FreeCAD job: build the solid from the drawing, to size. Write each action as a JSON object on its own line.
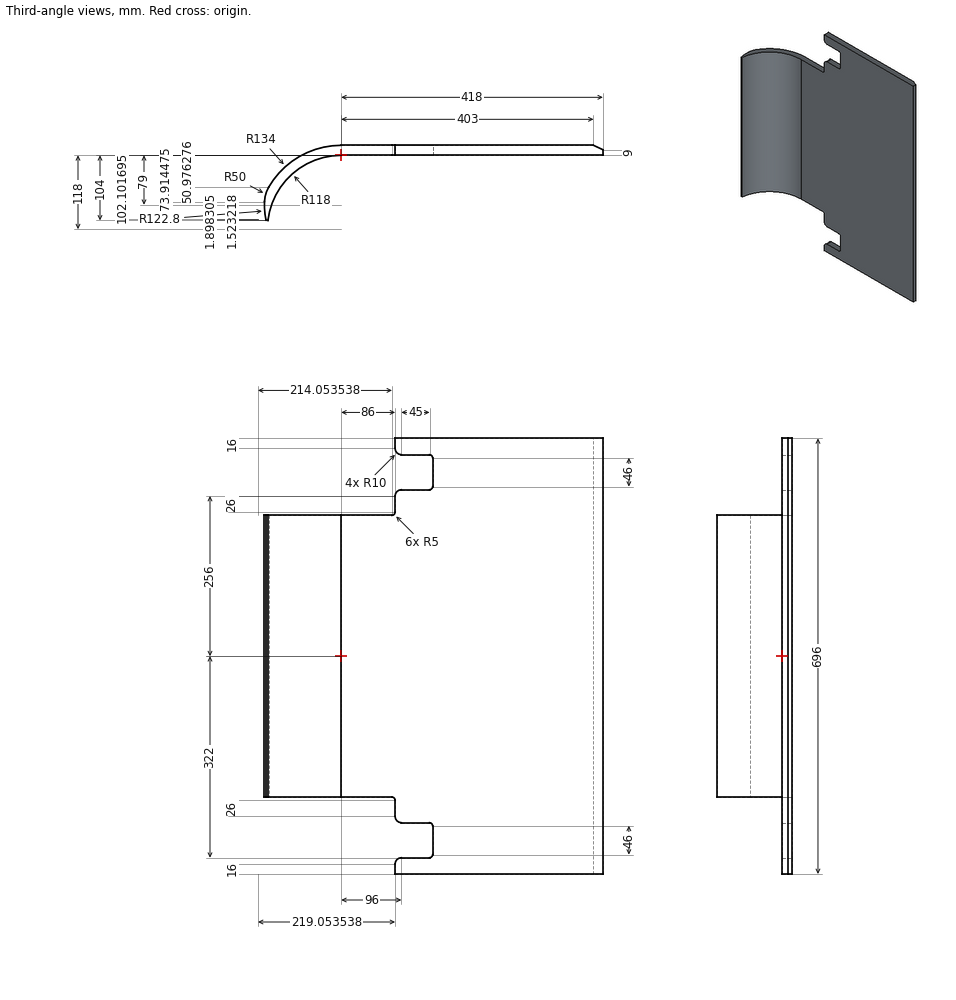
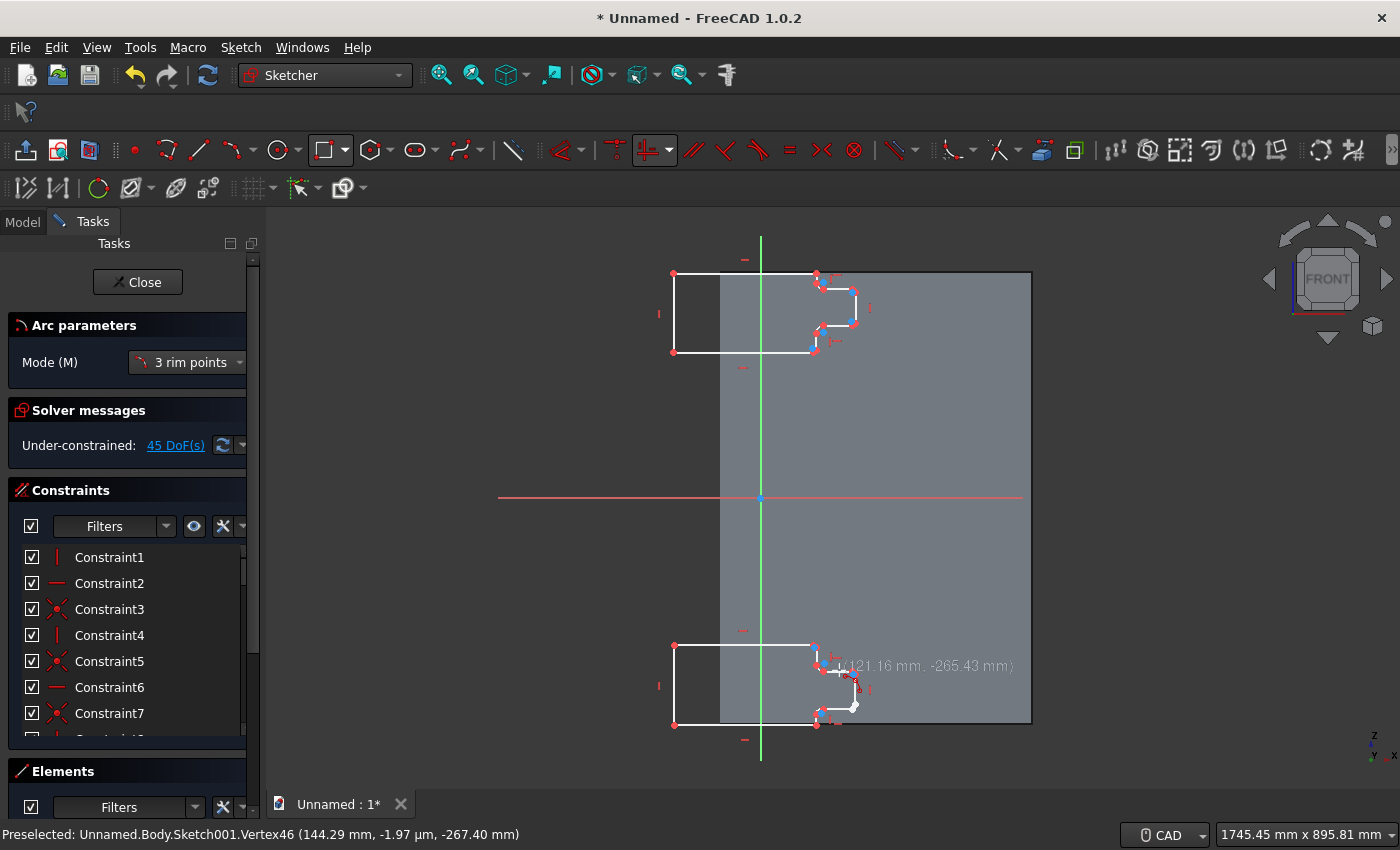
{"action": "scroll", "coordinate": [856, 704], "scroll_direction": "up", "scroll_amount": 7}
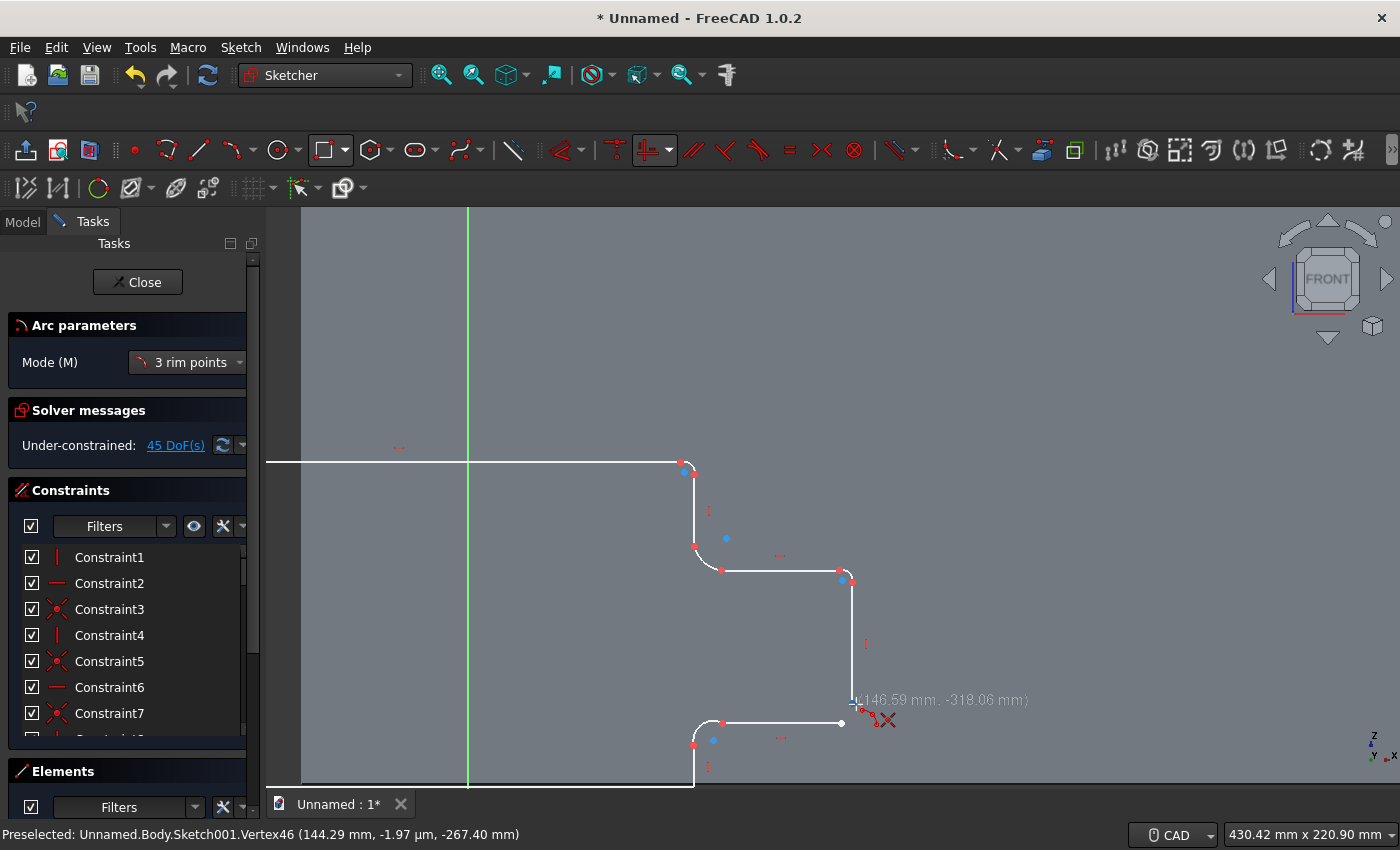
{"action": "left_click", "coordinate": [852, 704]}
{"action": "left_click", "coordinate": [841, 723]}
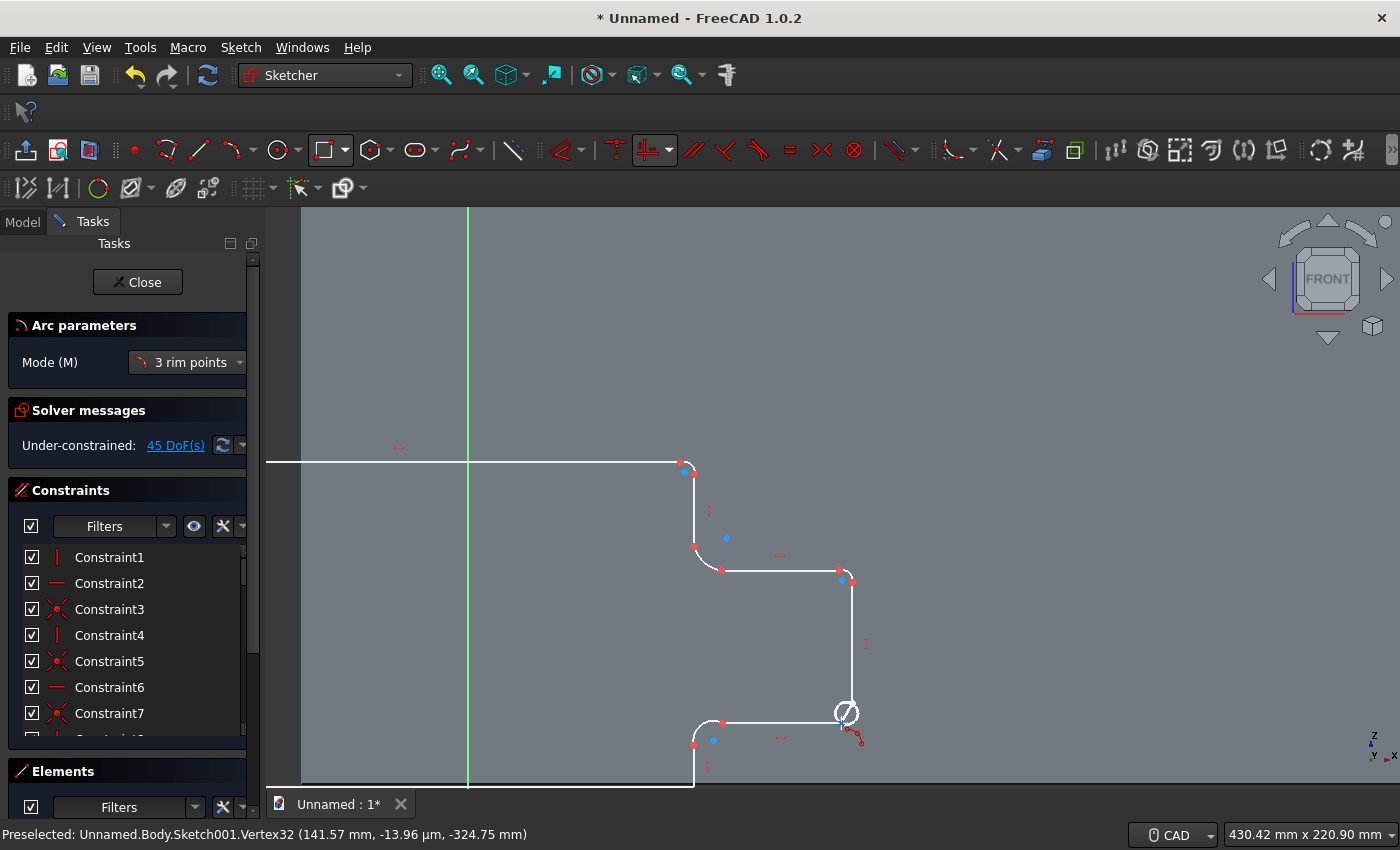
{"action": "scroll", "coordinate": [849, 712], "scroll_direction": "up", "scroll_amount": 8}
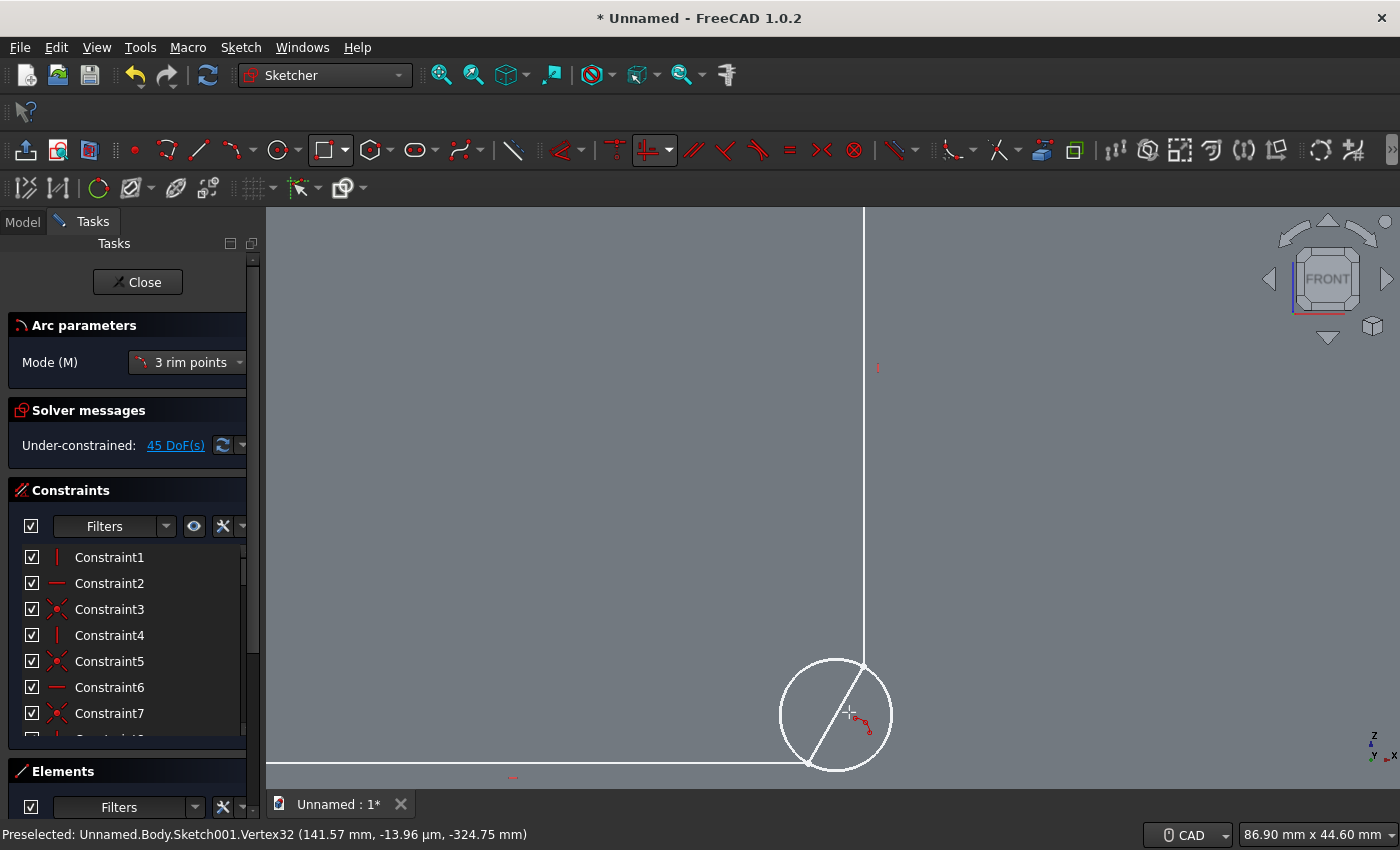
{"action": "left_click", "coordinate": [847, 708]}
{"action": "key", "text": "Escape"}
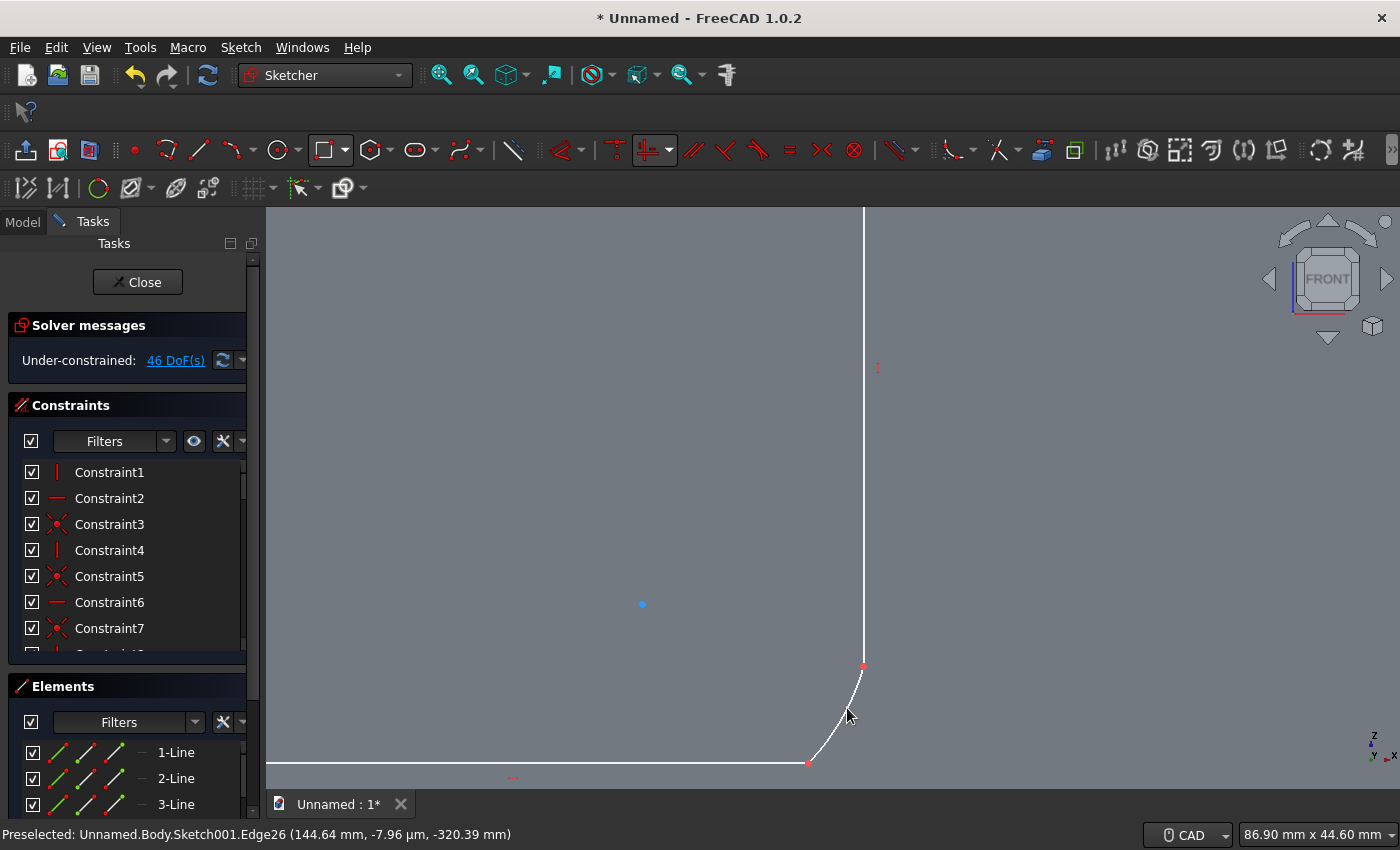
{"action": "scroll", "coordinate": [855, 706], "scroll_direction": "down", "scroll_amount": 15}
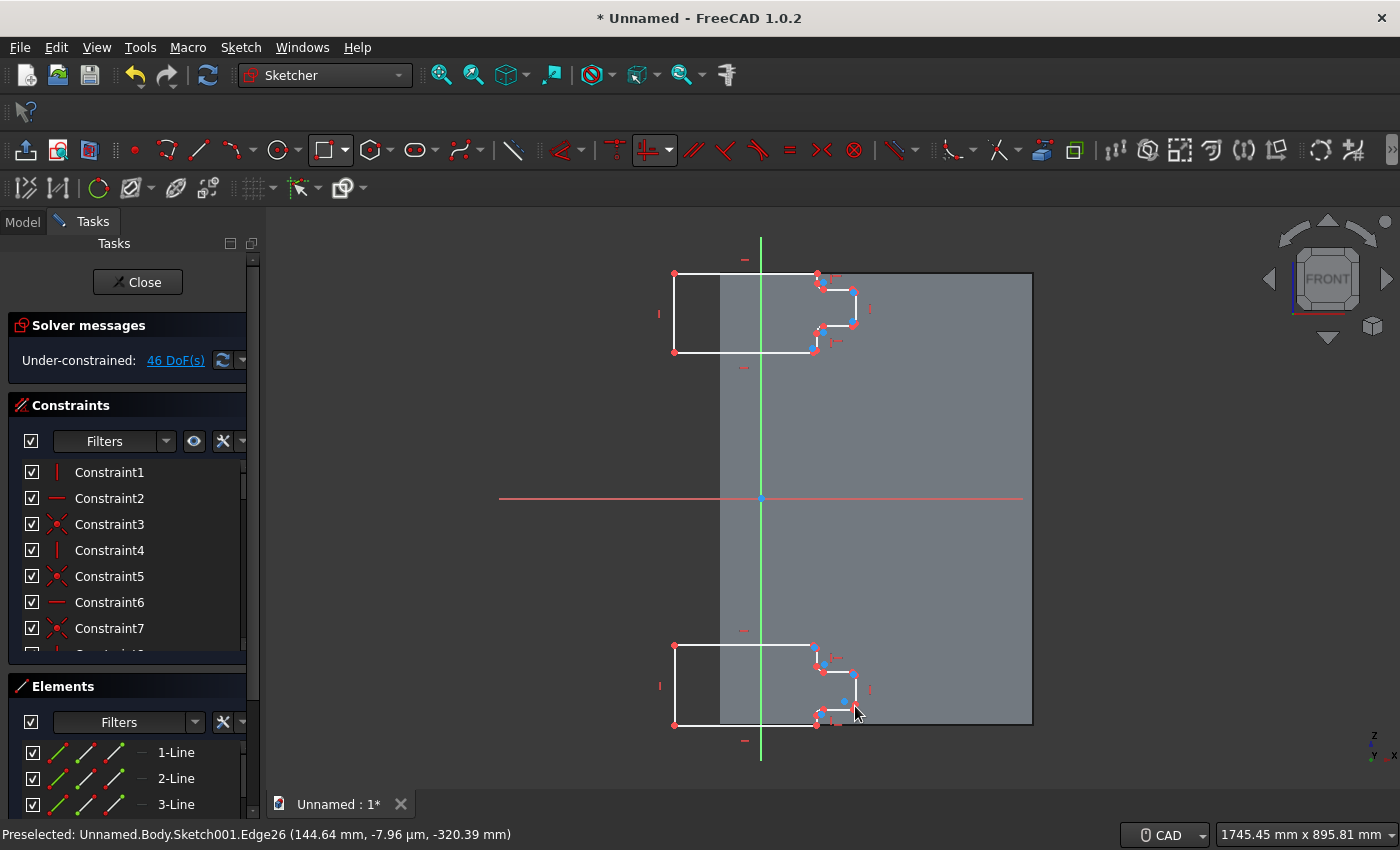
{"action": "scroll", "coordinate": [817, 339], "scroll_direction": "up", "scroll_amount": 5}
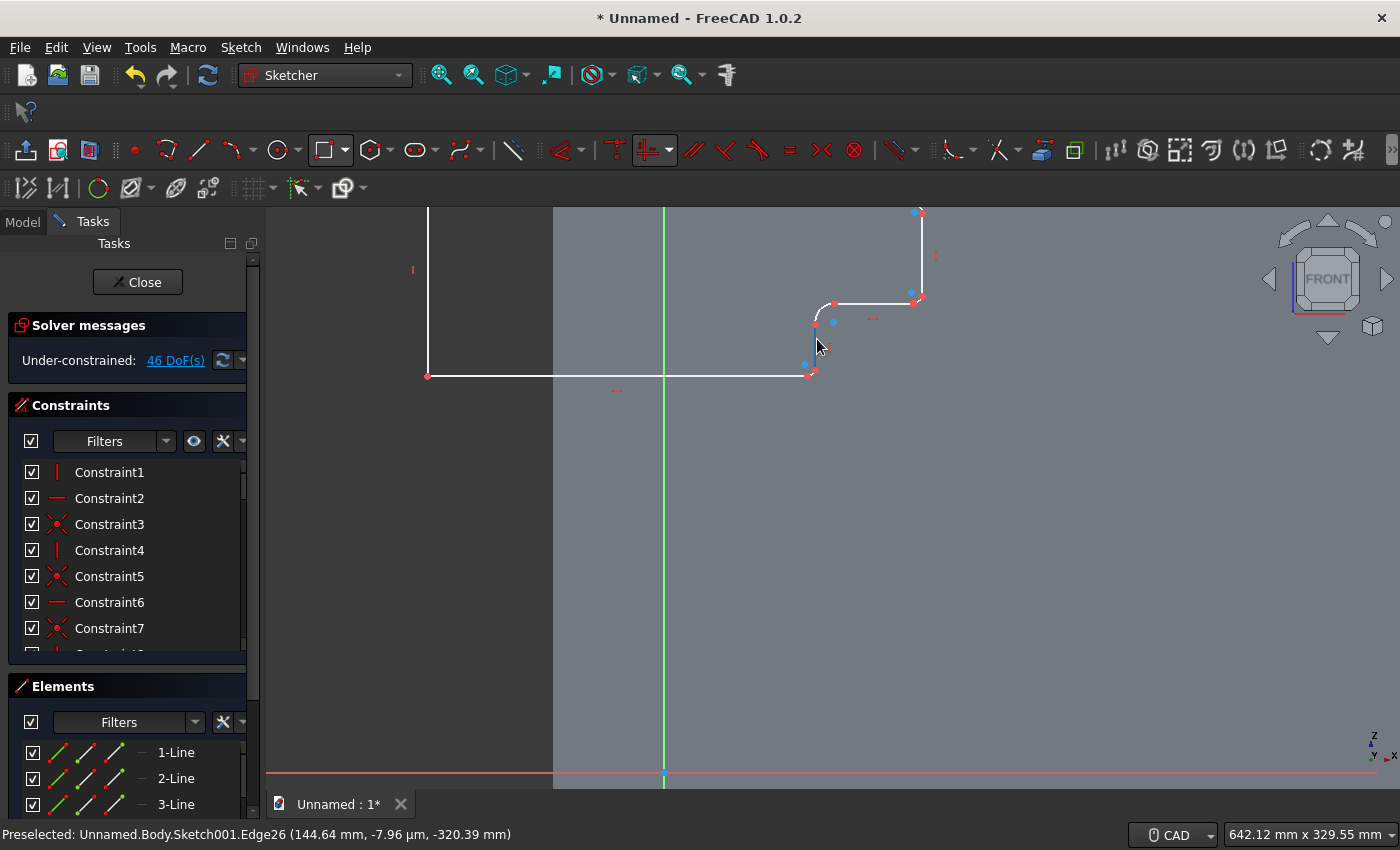
{"action": "left_click", "coordinate": [815, 338]}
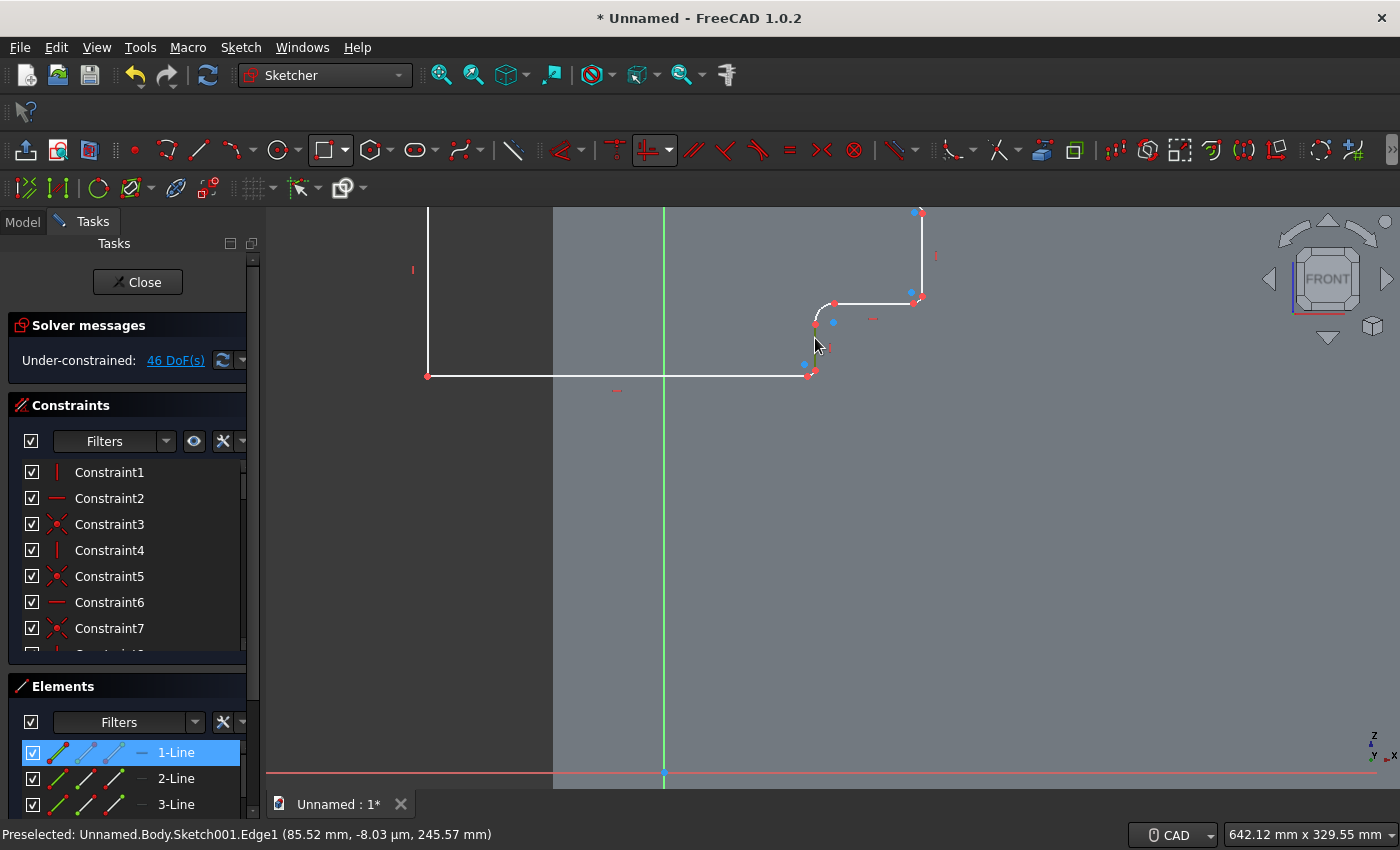
{"action": "scroll", "coordinate": [812, 374], "scroll_direction": "up", "scroll_amount": 6}